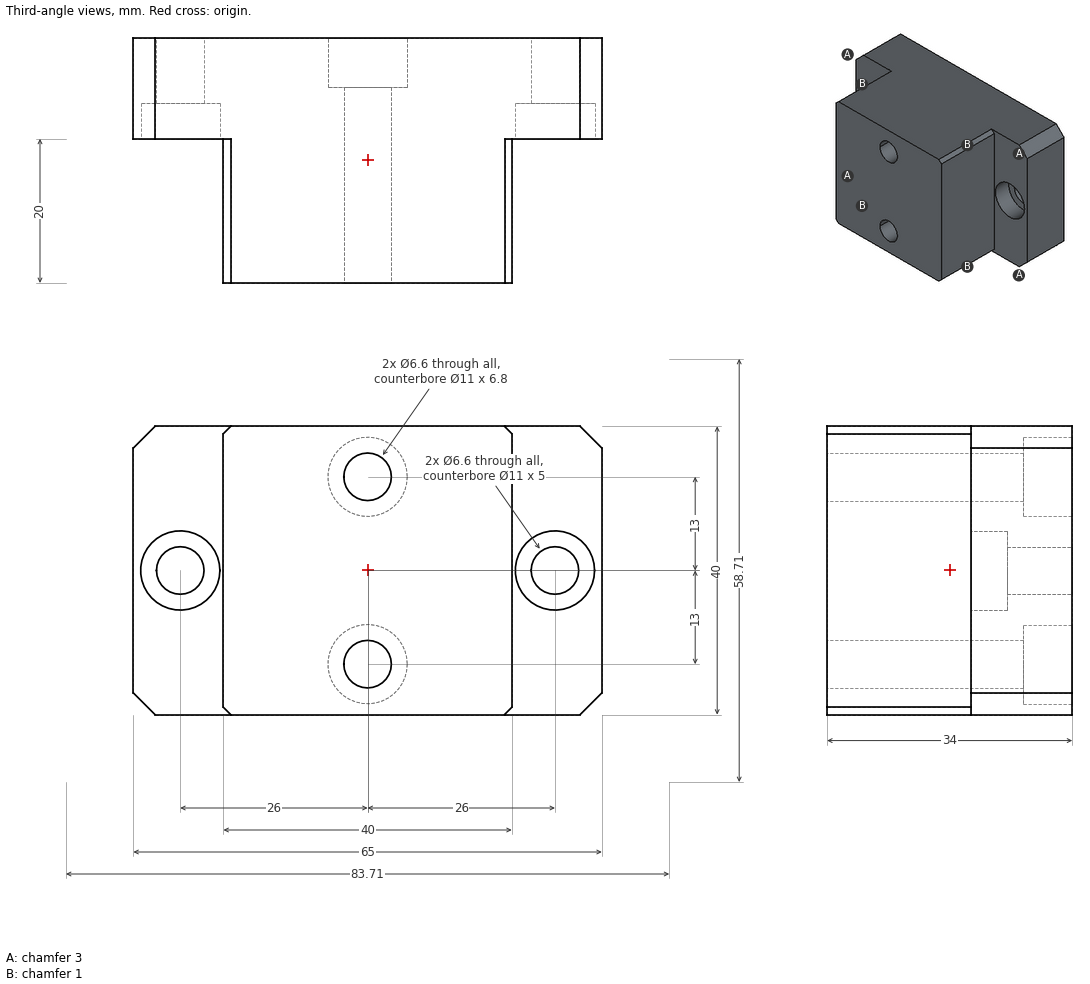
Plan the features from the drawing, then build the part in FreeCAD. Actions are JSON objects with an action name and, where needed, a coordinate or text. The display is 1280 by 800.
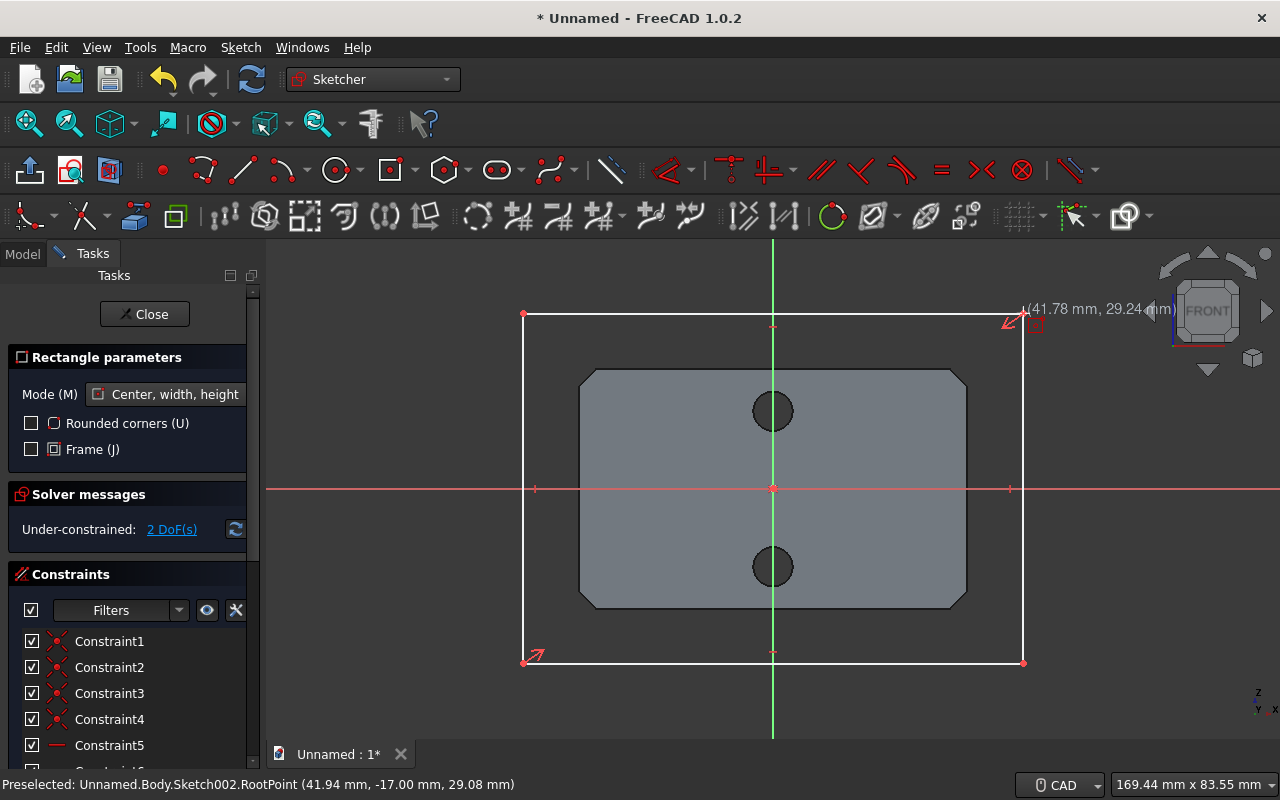
{"action": "left_click", "coordinate": [773, 489]}
{"action": "left_click", "coordinate": [893, 369]}
{"action": "key", "text": "Escape"}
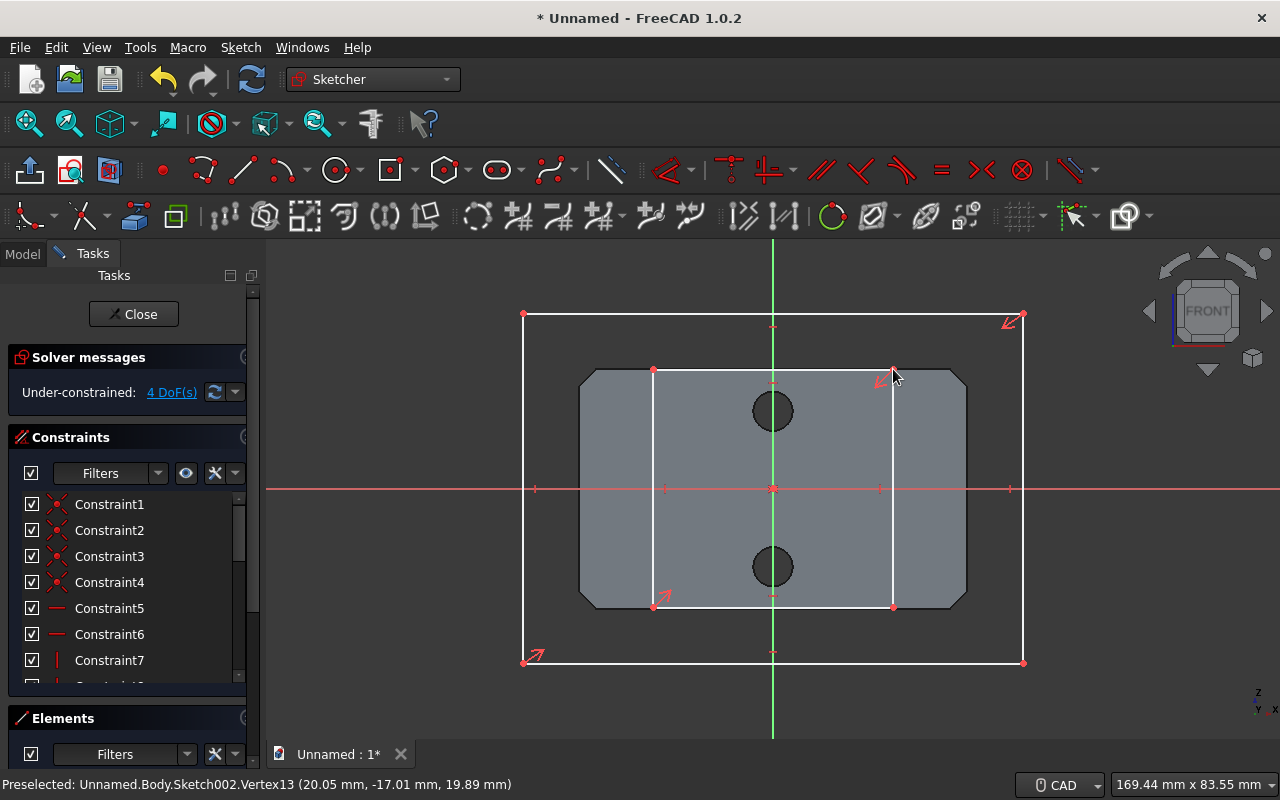
{"action": "left_click", "coordinate": [666, 170]}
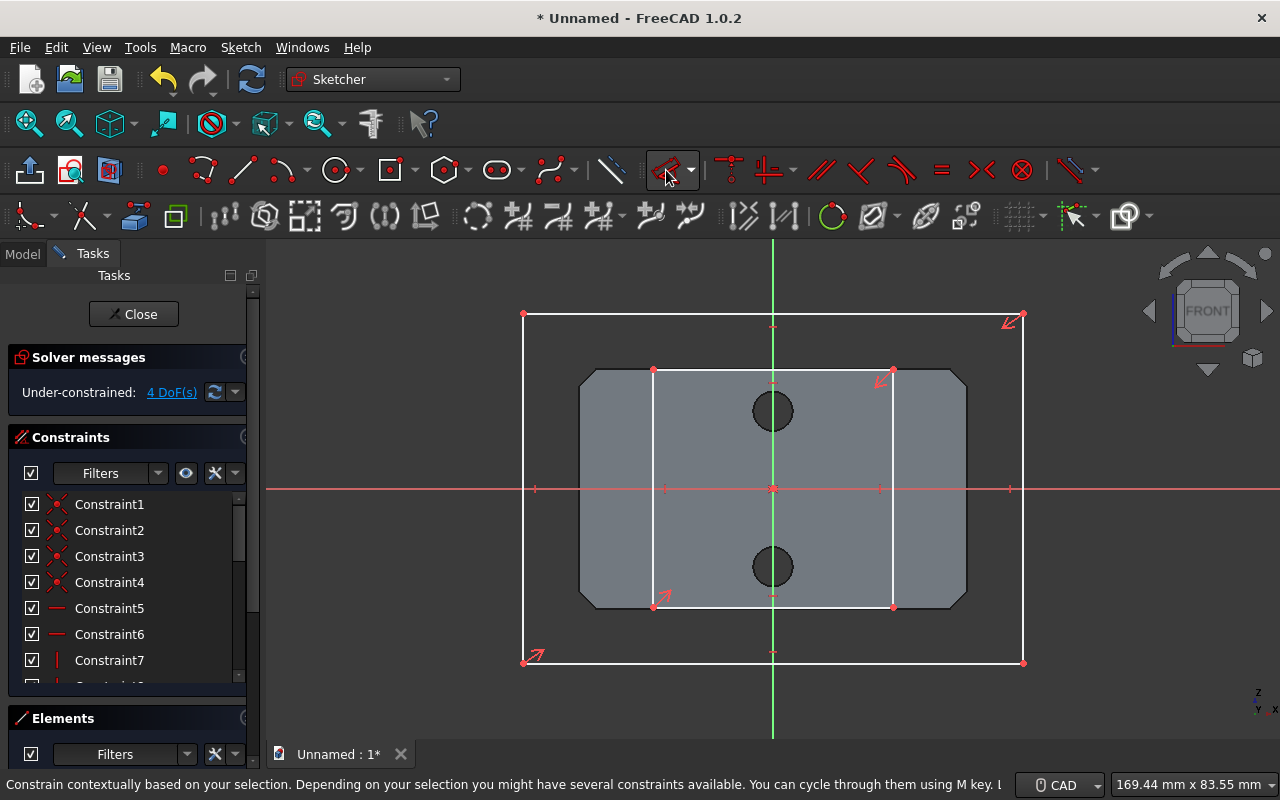
{"action": "left_click", "coordinate": [725, 608]}
{"action": "left_click", "coordinate": [718, 642]}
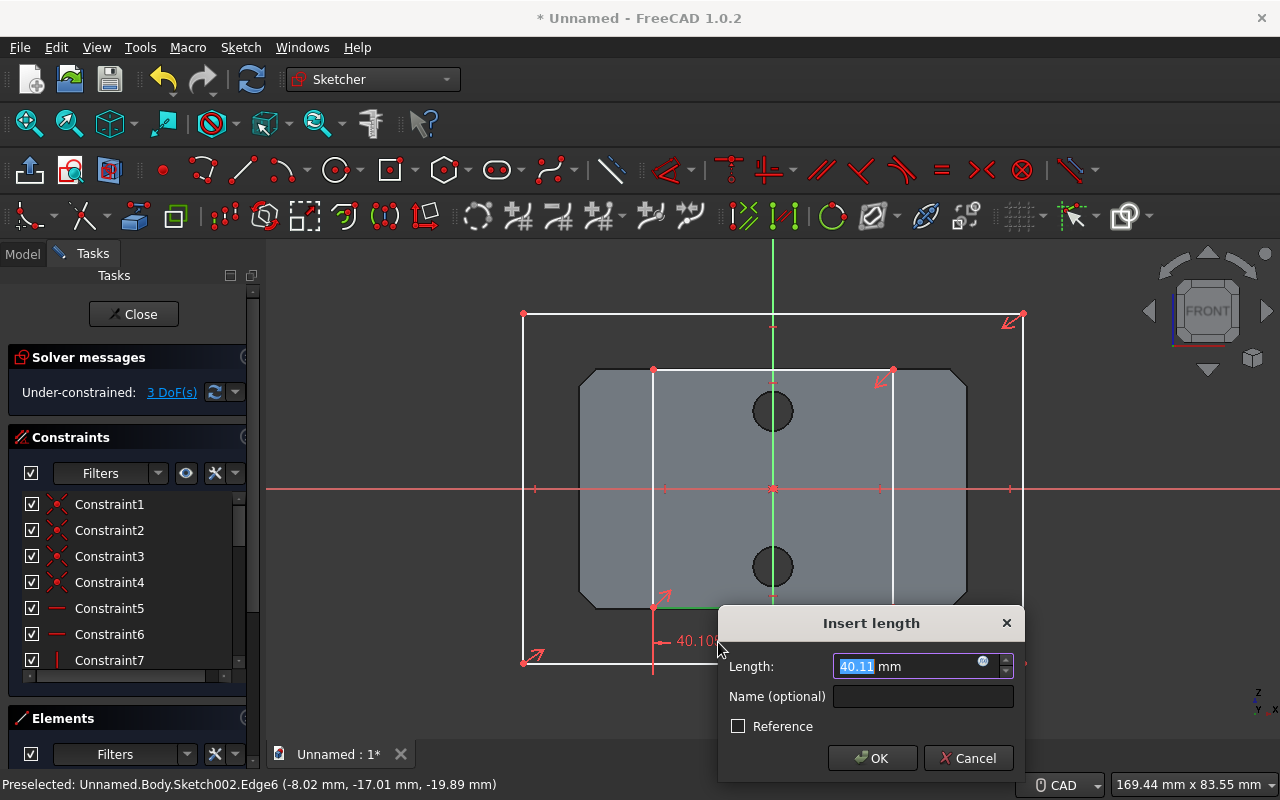
{"action": "type", "text": "40"}
{"action": "key", "text": "Return"}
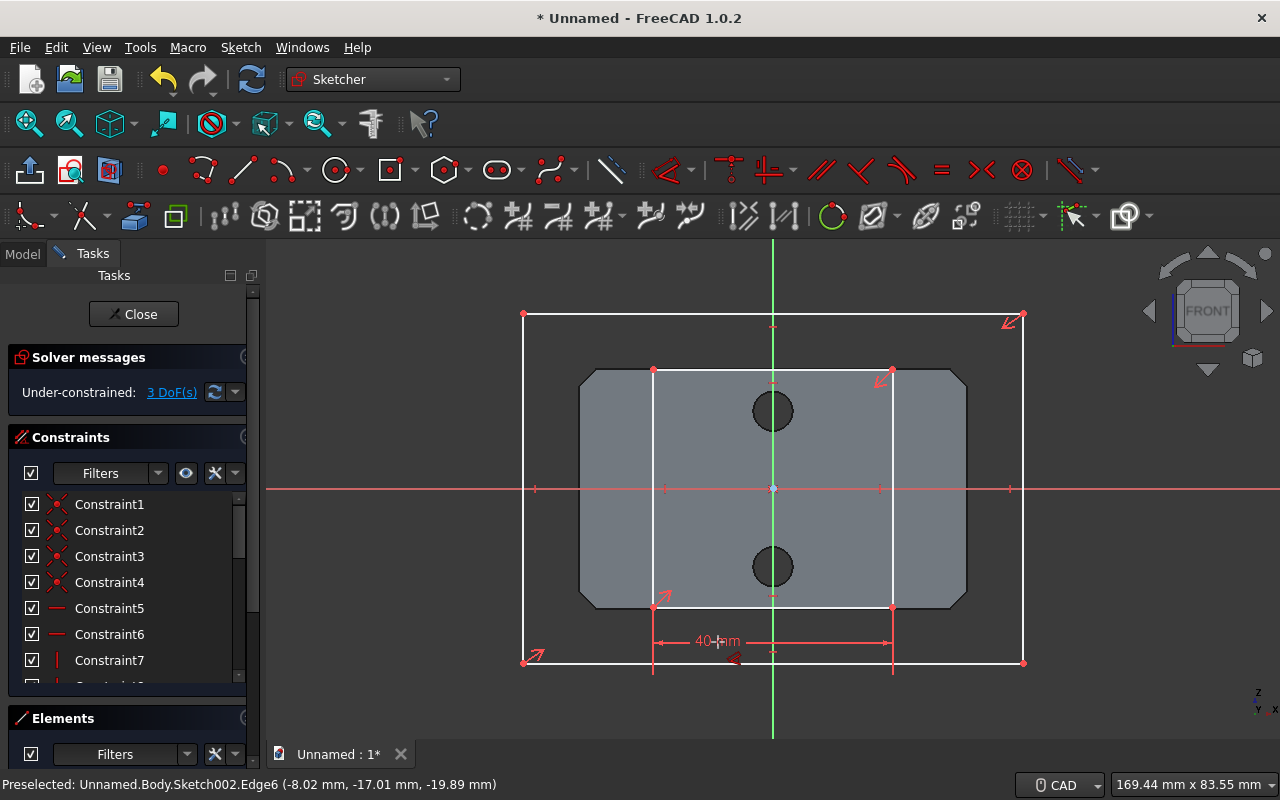
{"action": "left_click", "coordinate": [893, 537]}
{"action": "left_click", "coordinate": [927, 434]}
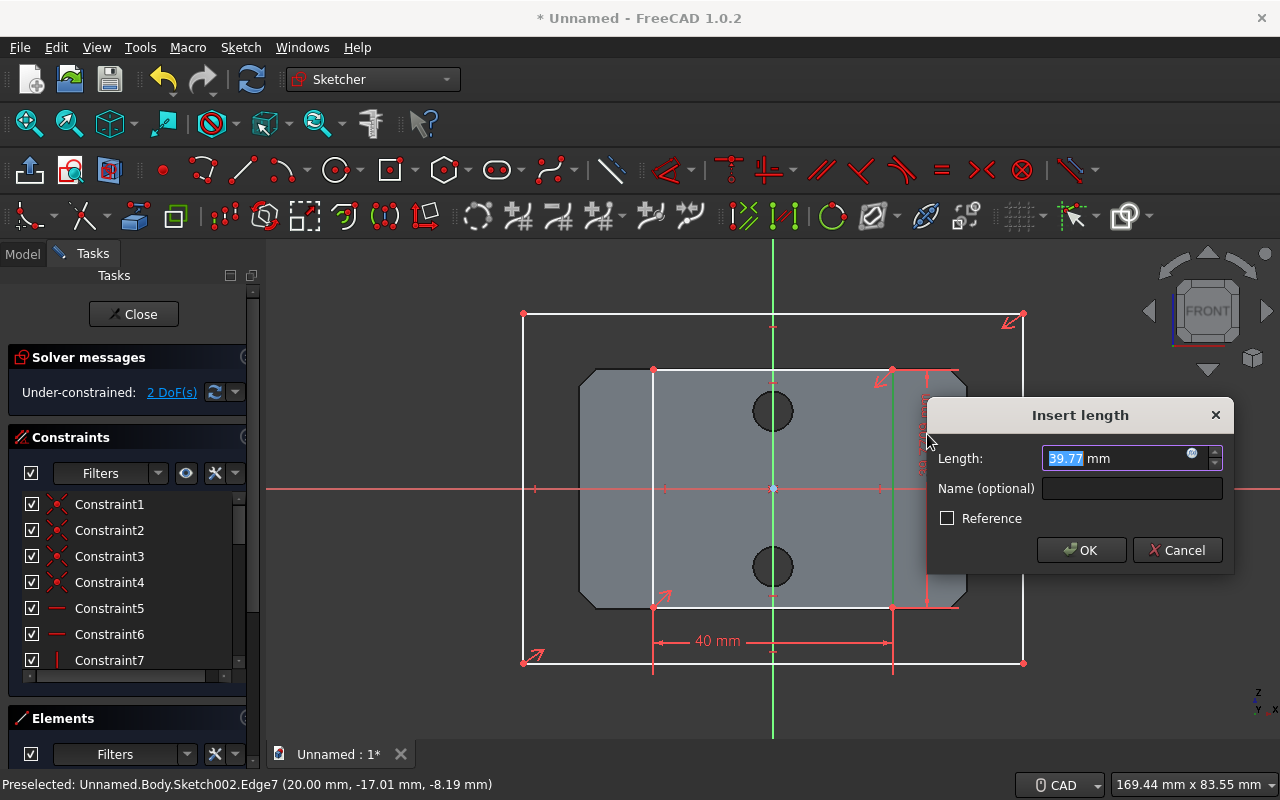
{"action": "type", "text": "40"}
{"action": "key", "text": "Return"}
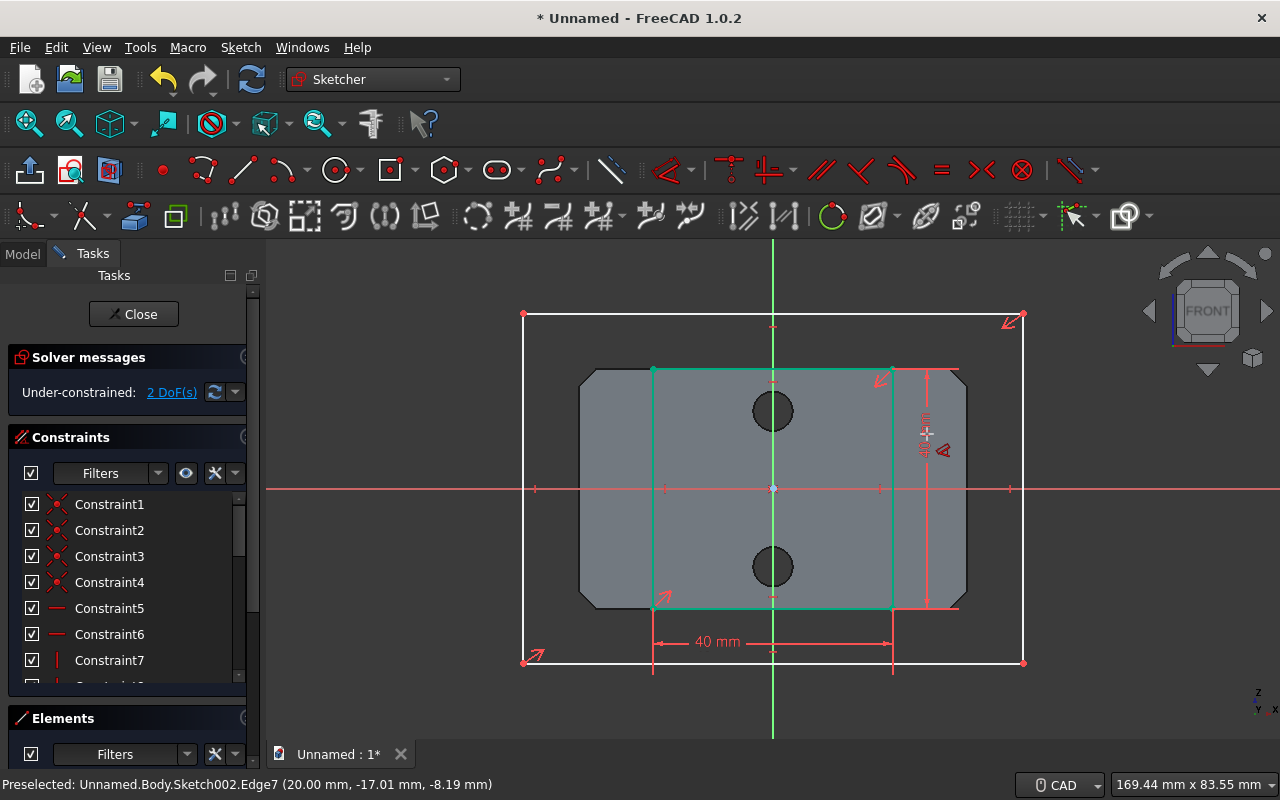
{"action": "left_click", "coordinate": [673, 664]}
{"action": "left_click", "coordinate": [658, 698]}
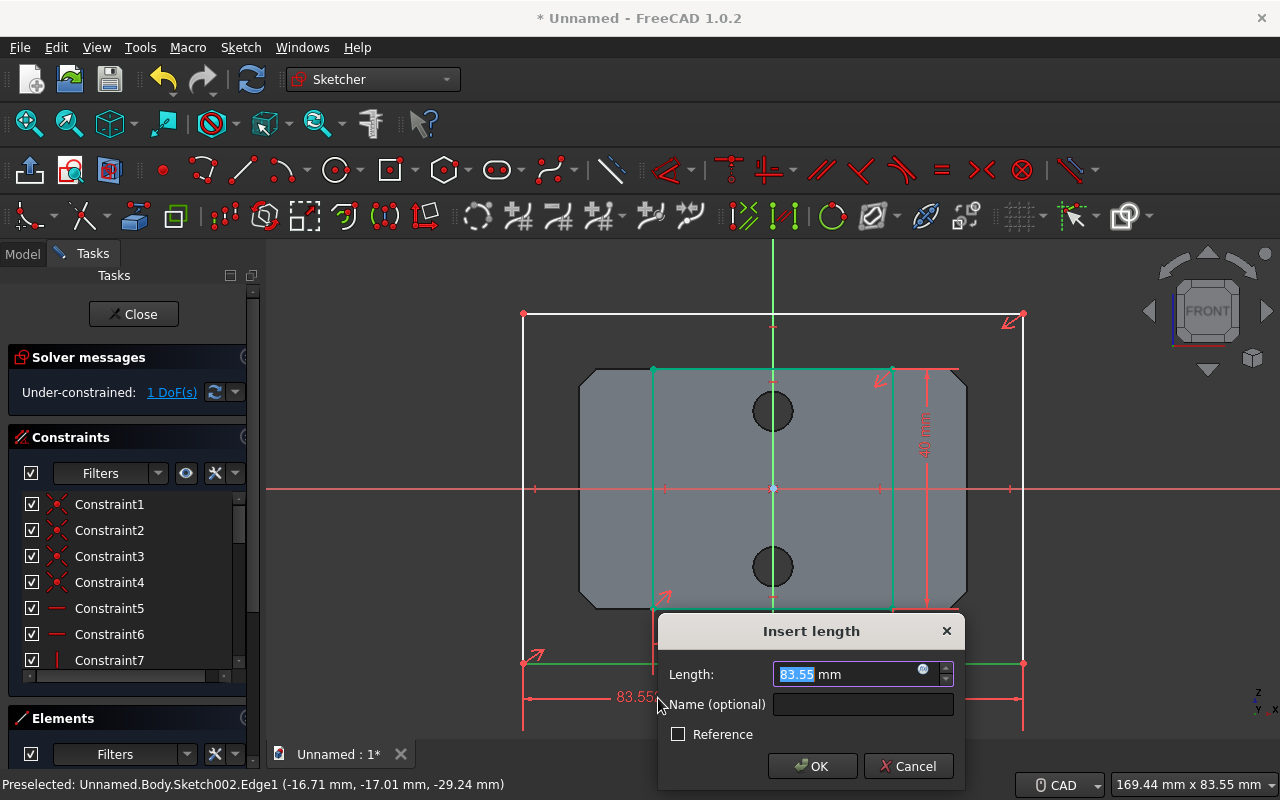
{"action": "type", "text": "83.71"}
{"action": "key", "text": "Return"}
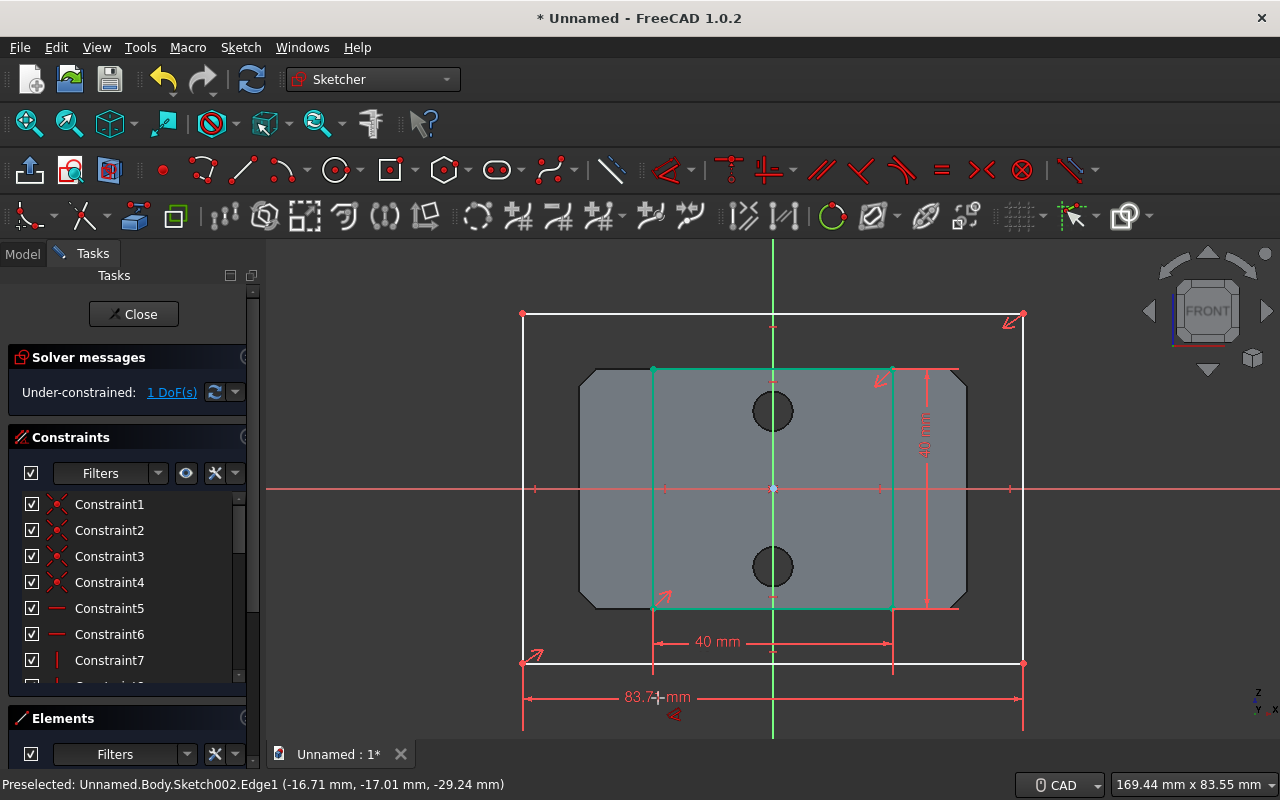
{"action": "left_click", "coordinate": [1023, 559]}
{"action": "left_click", "coordinate": [1057, 408]}